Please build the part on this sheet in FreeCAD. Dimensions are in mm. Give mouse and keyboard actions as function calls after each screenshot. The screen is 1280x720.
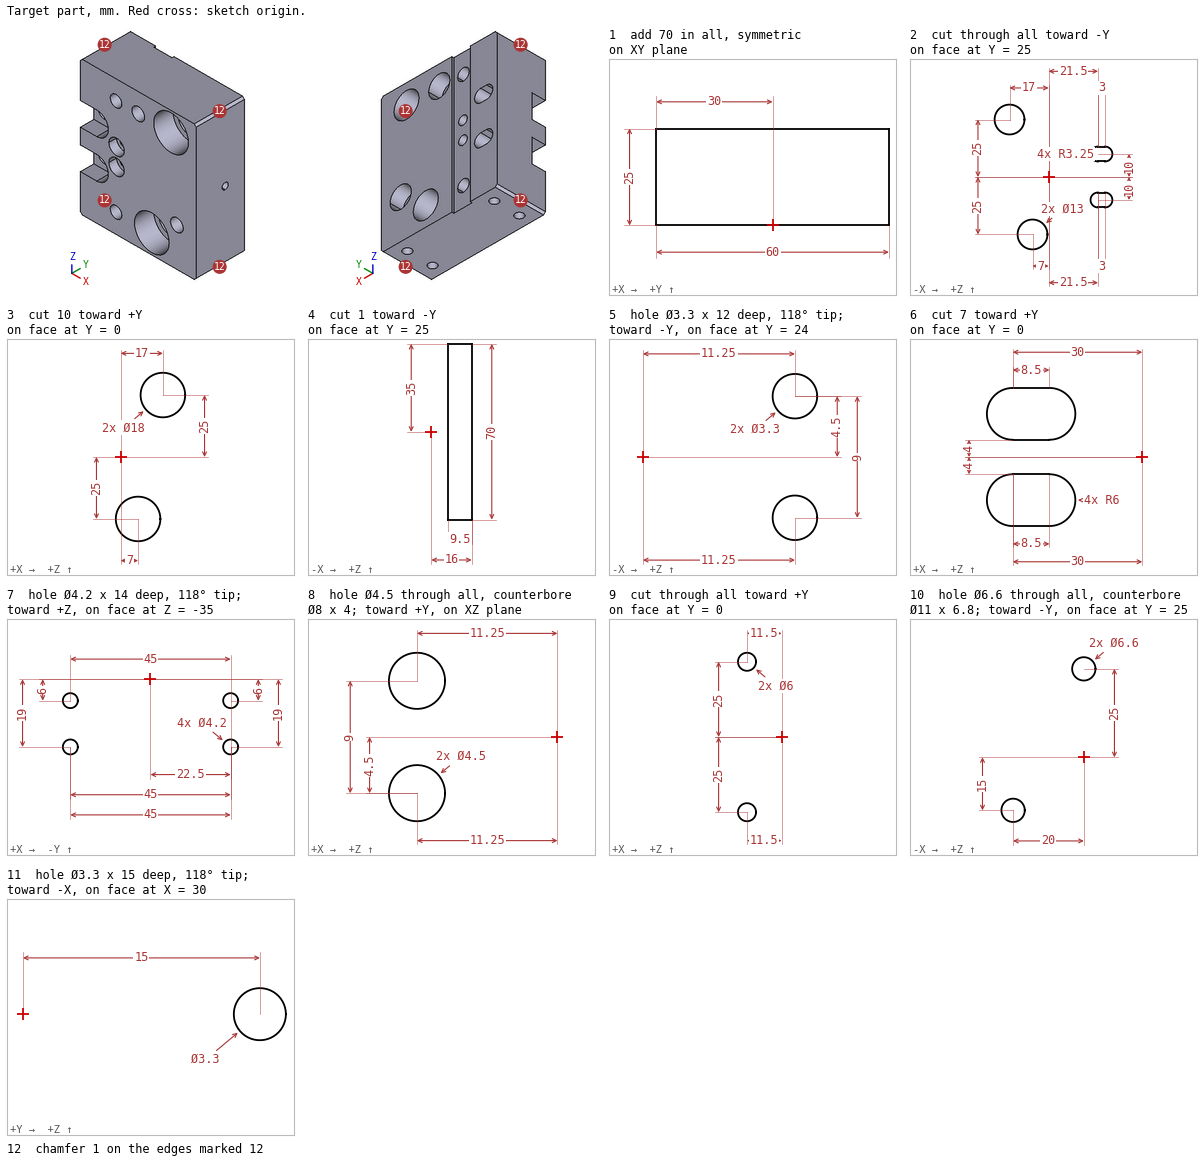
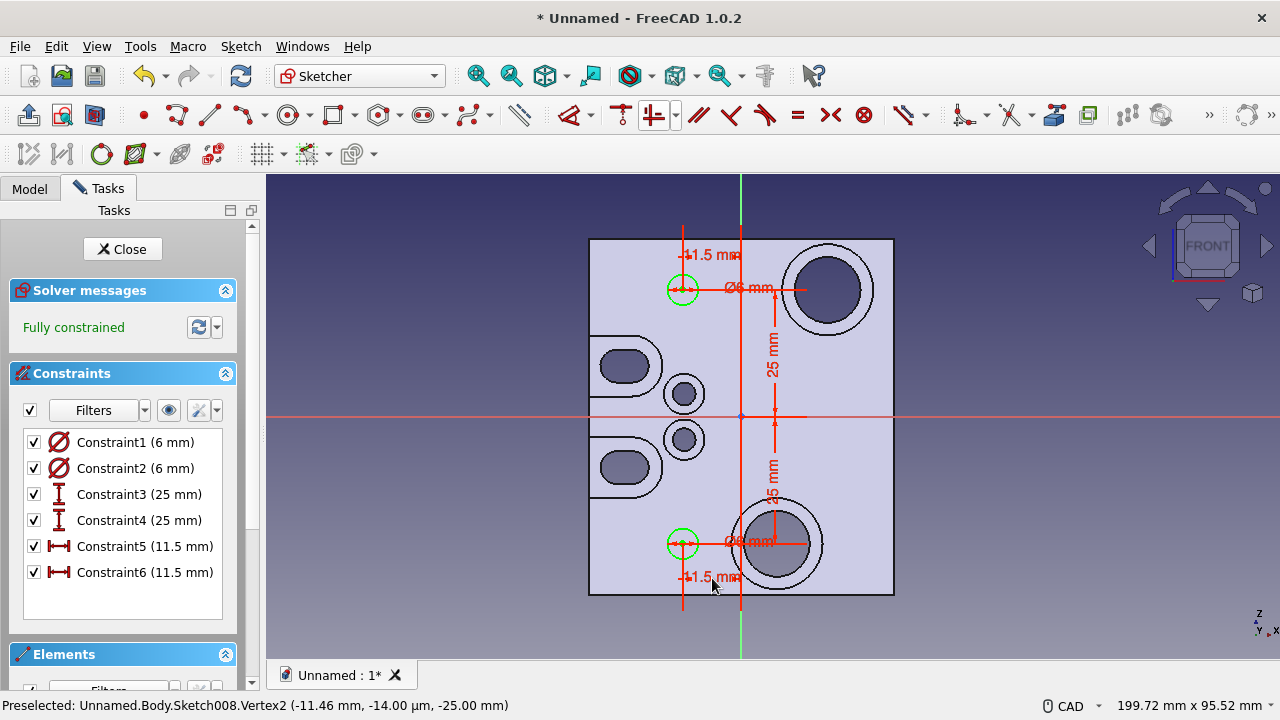
click(123, 249)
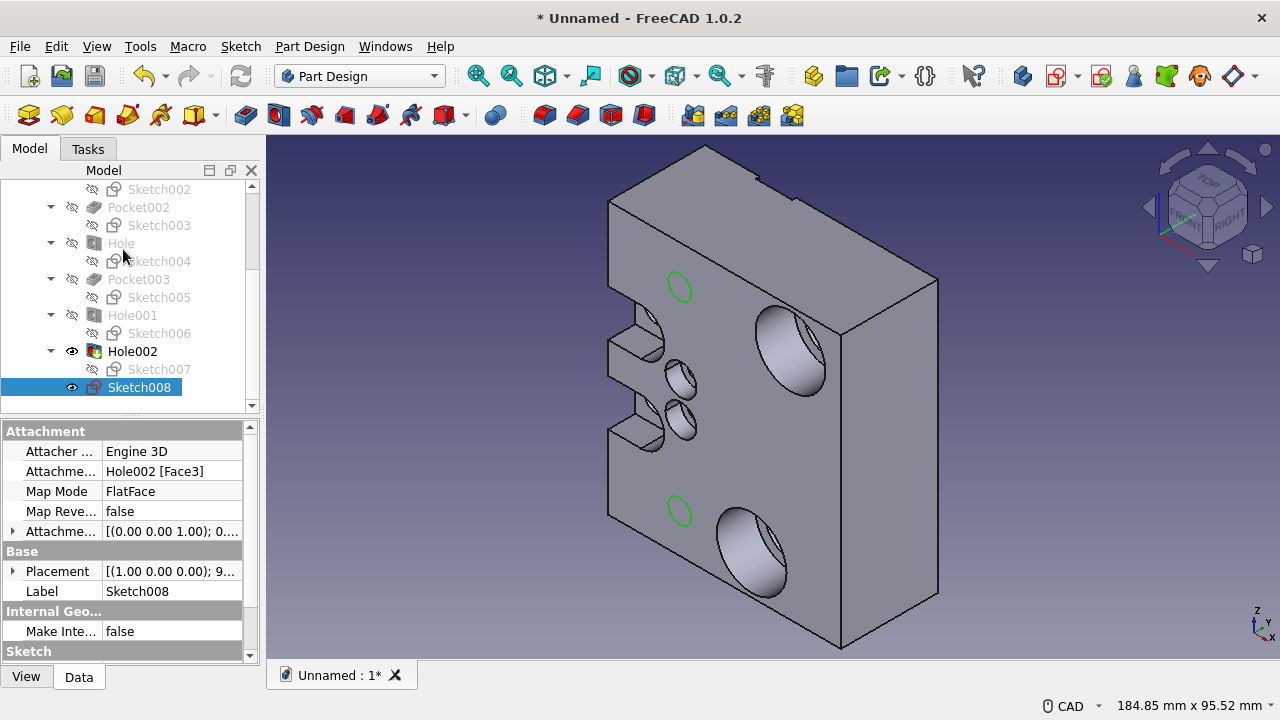
click(246, 116)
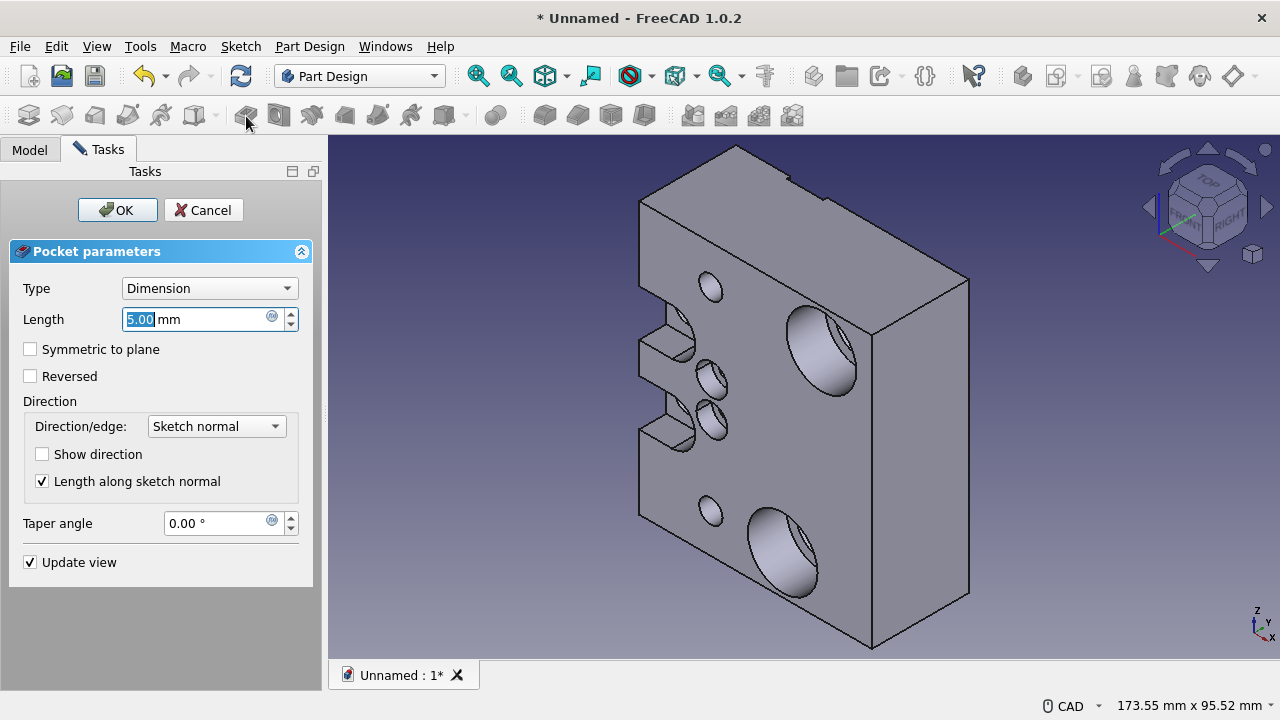
click(210, 288)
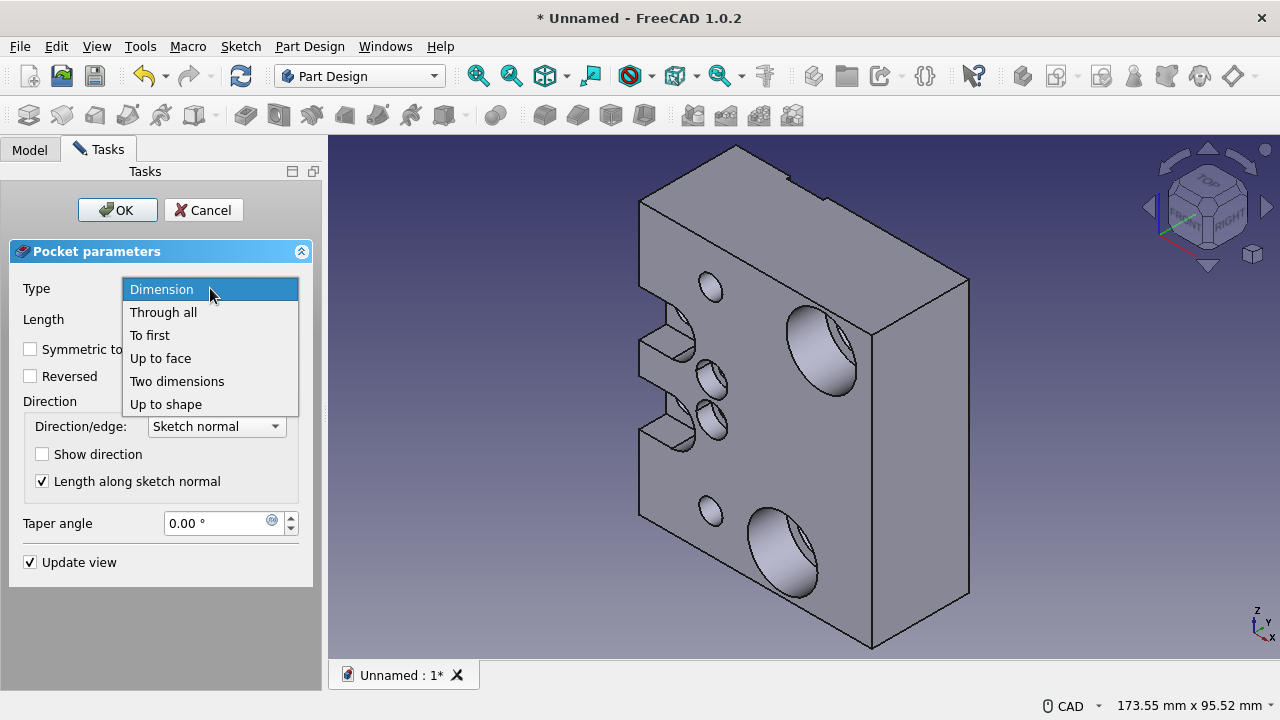
click(208, 312)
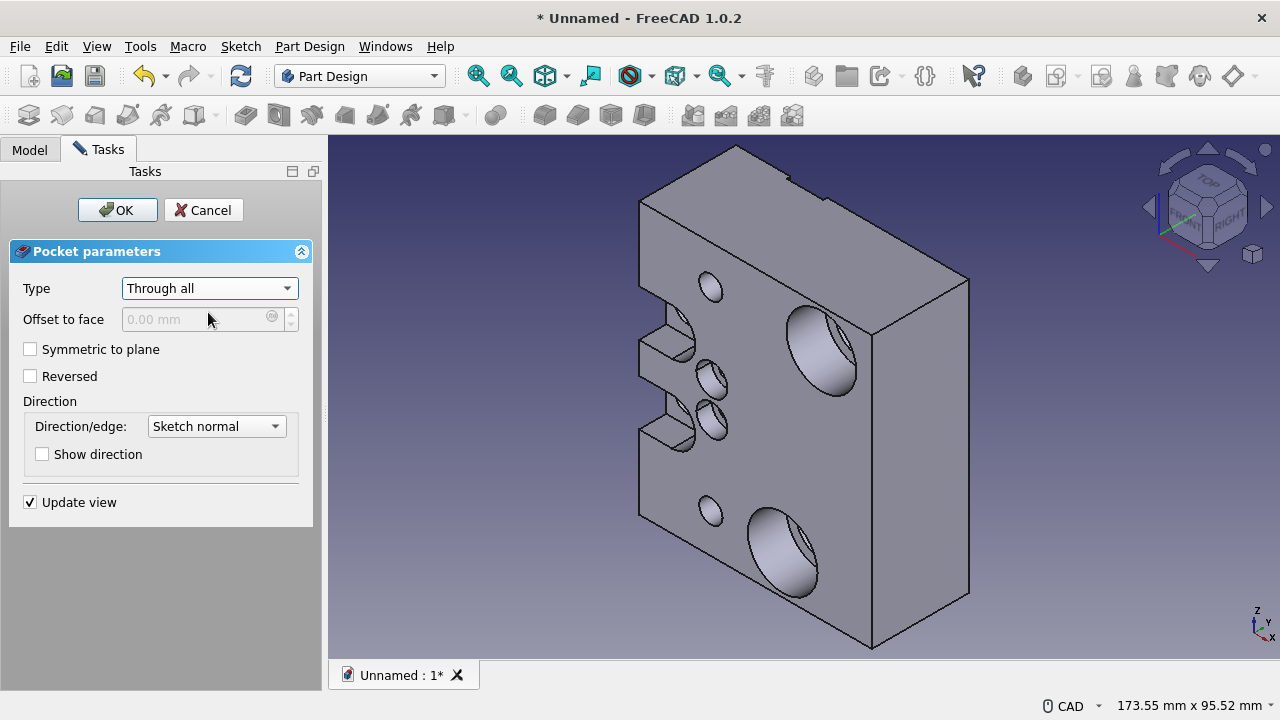
click(118, 210)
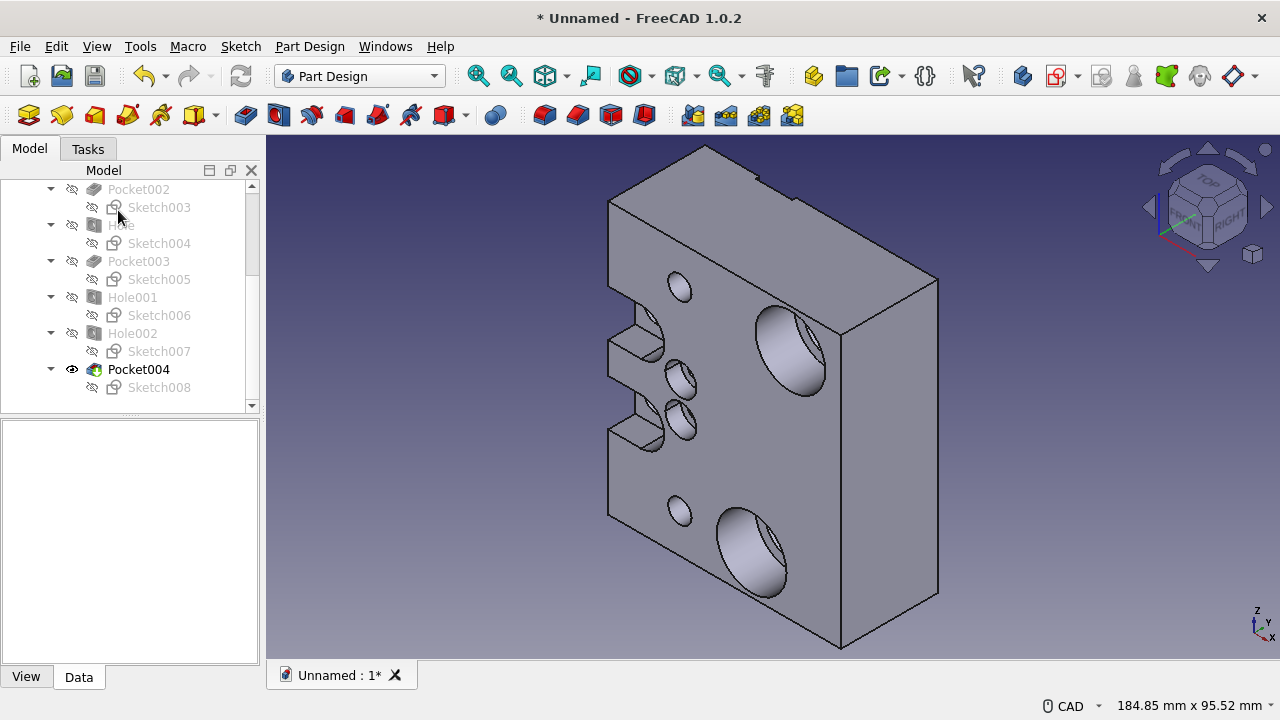
key(4)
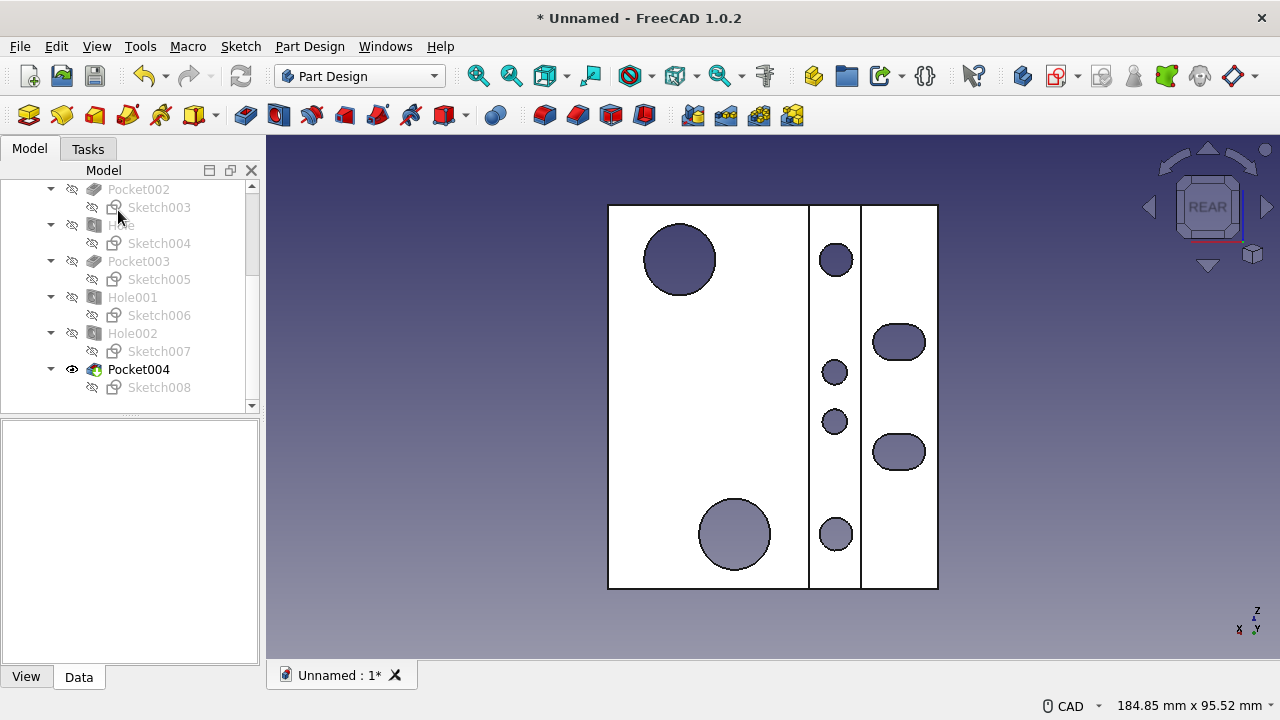
click(709, 396)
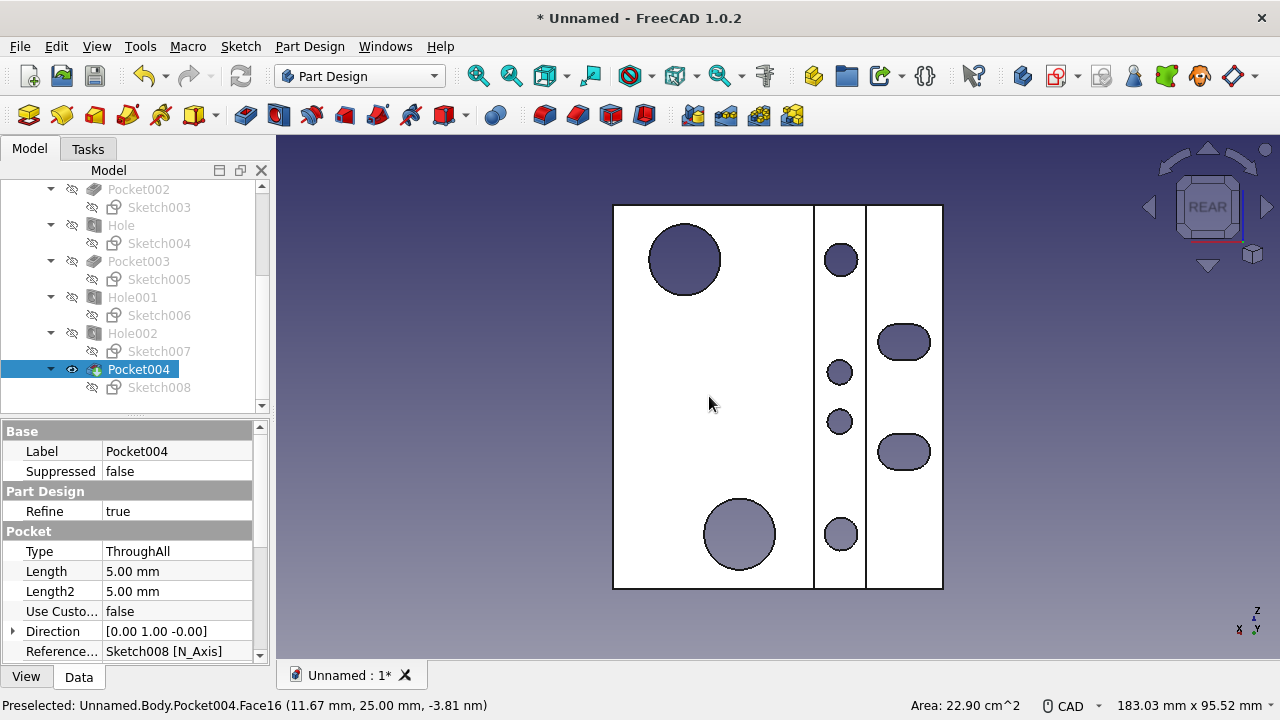
click(1056, 76)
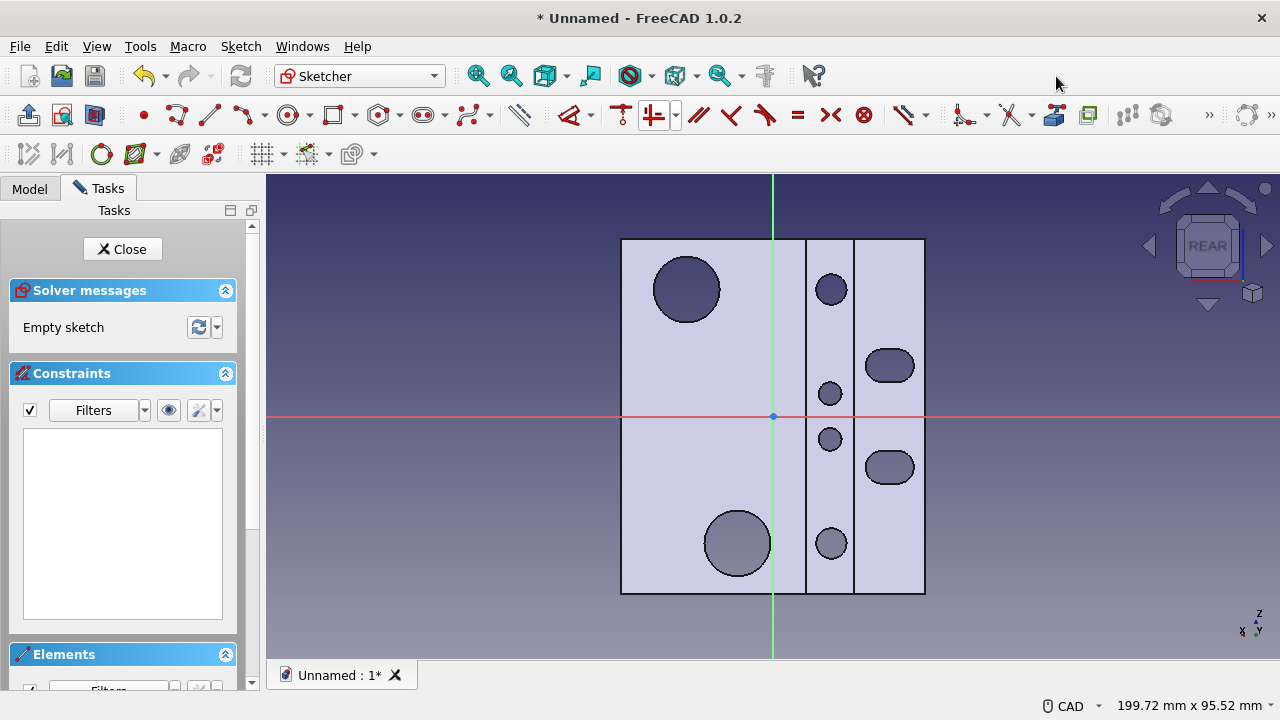
click(288, 116)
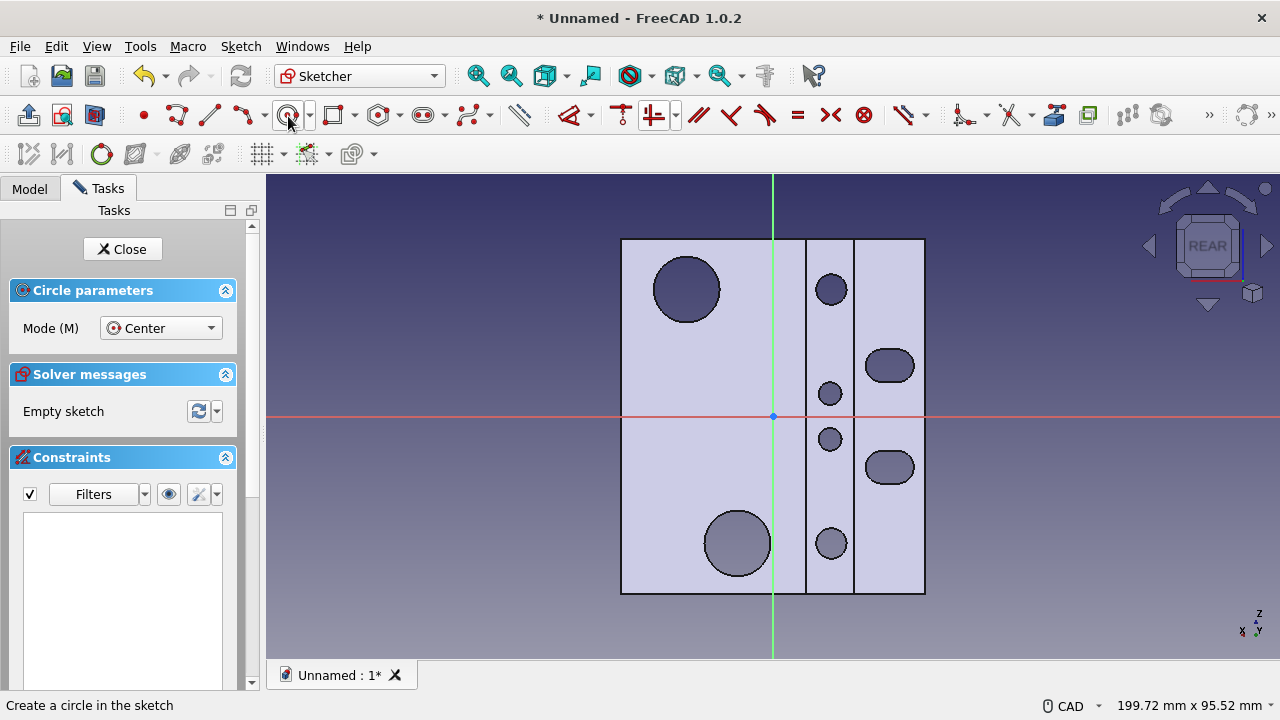
scroll(773, 290, up, 2)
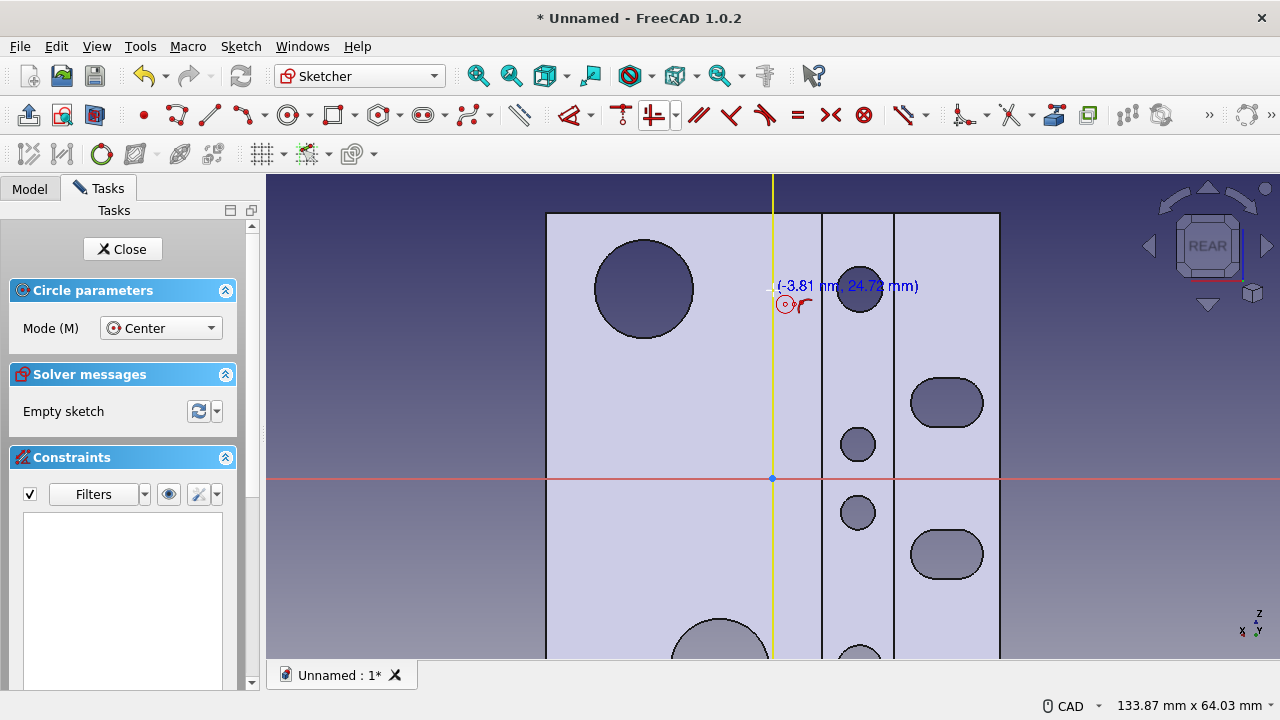
click(773, 289)
move(790, 272)